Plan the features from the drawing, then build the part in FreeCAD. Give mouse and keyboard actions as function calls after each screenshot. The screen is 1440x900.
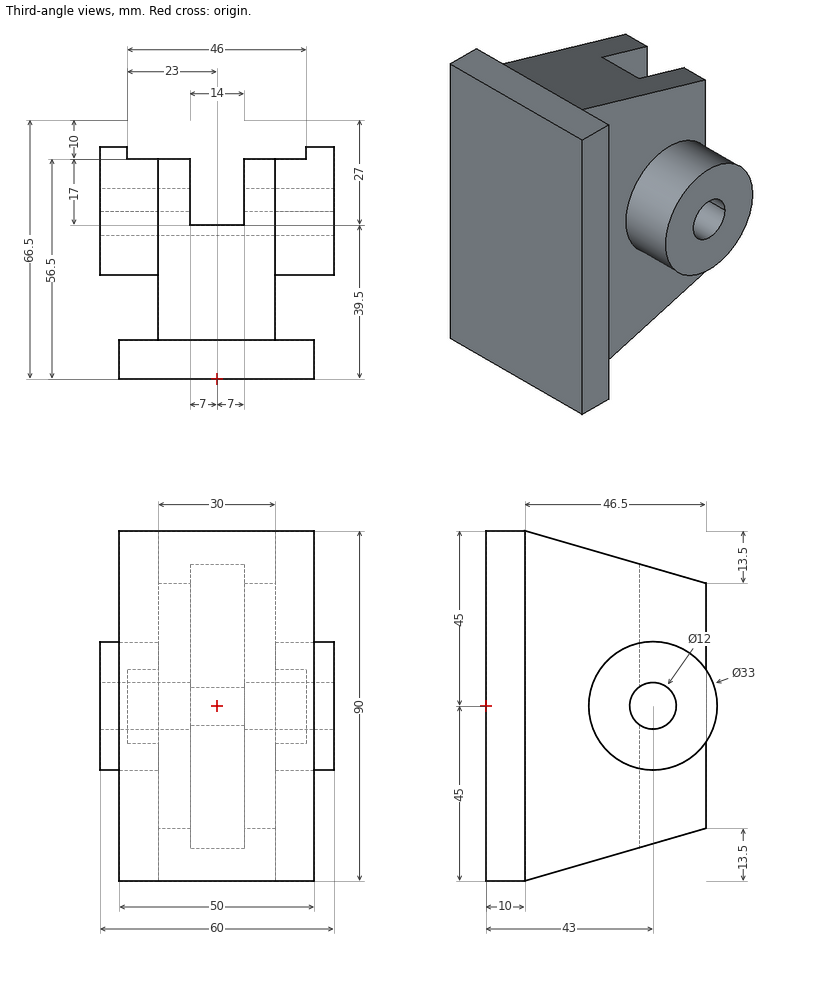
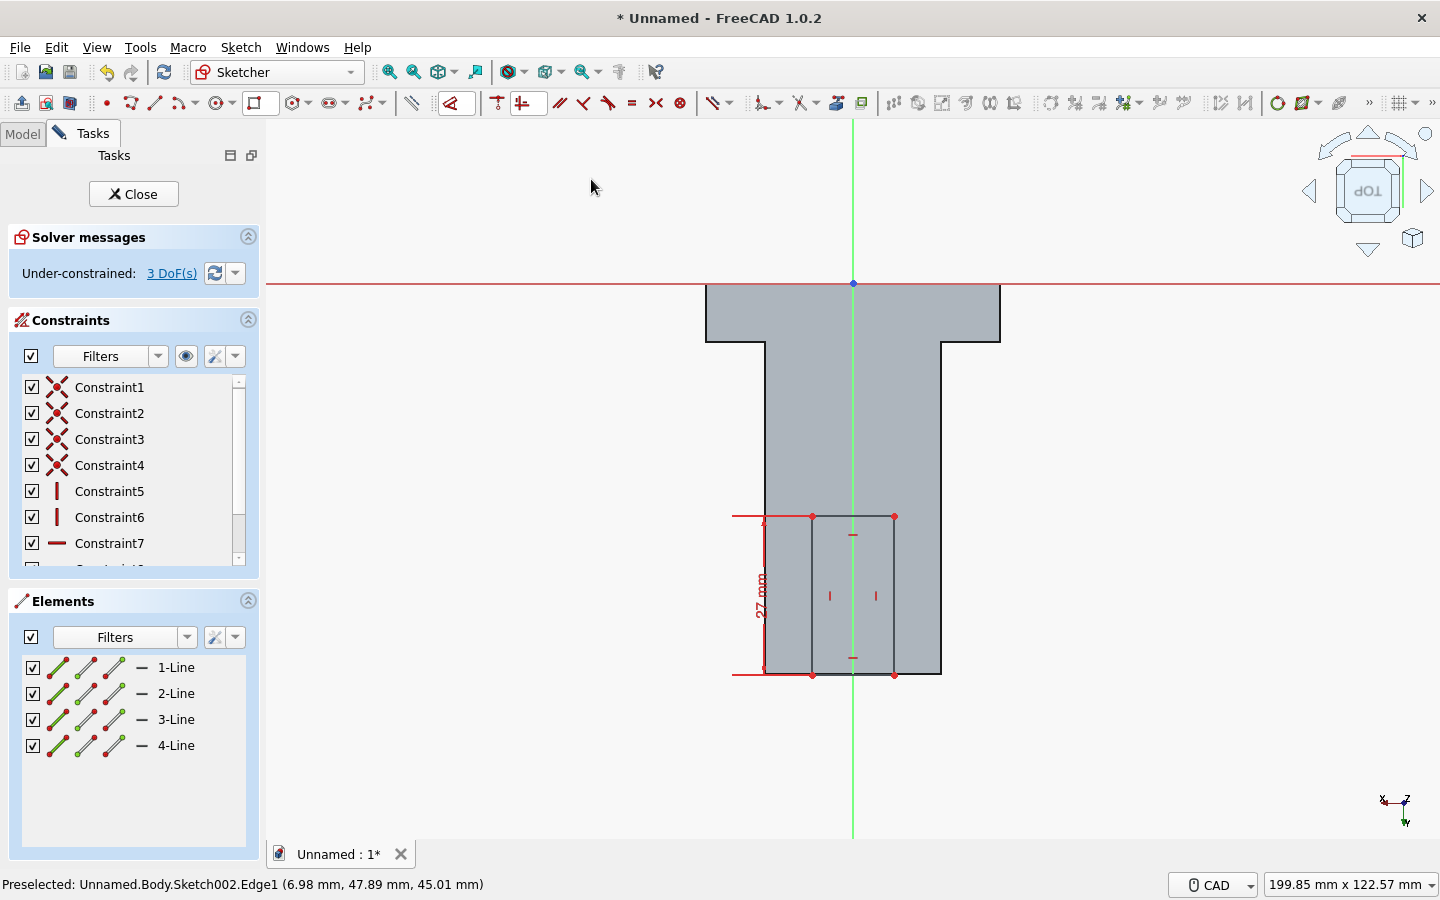
click(837, 675)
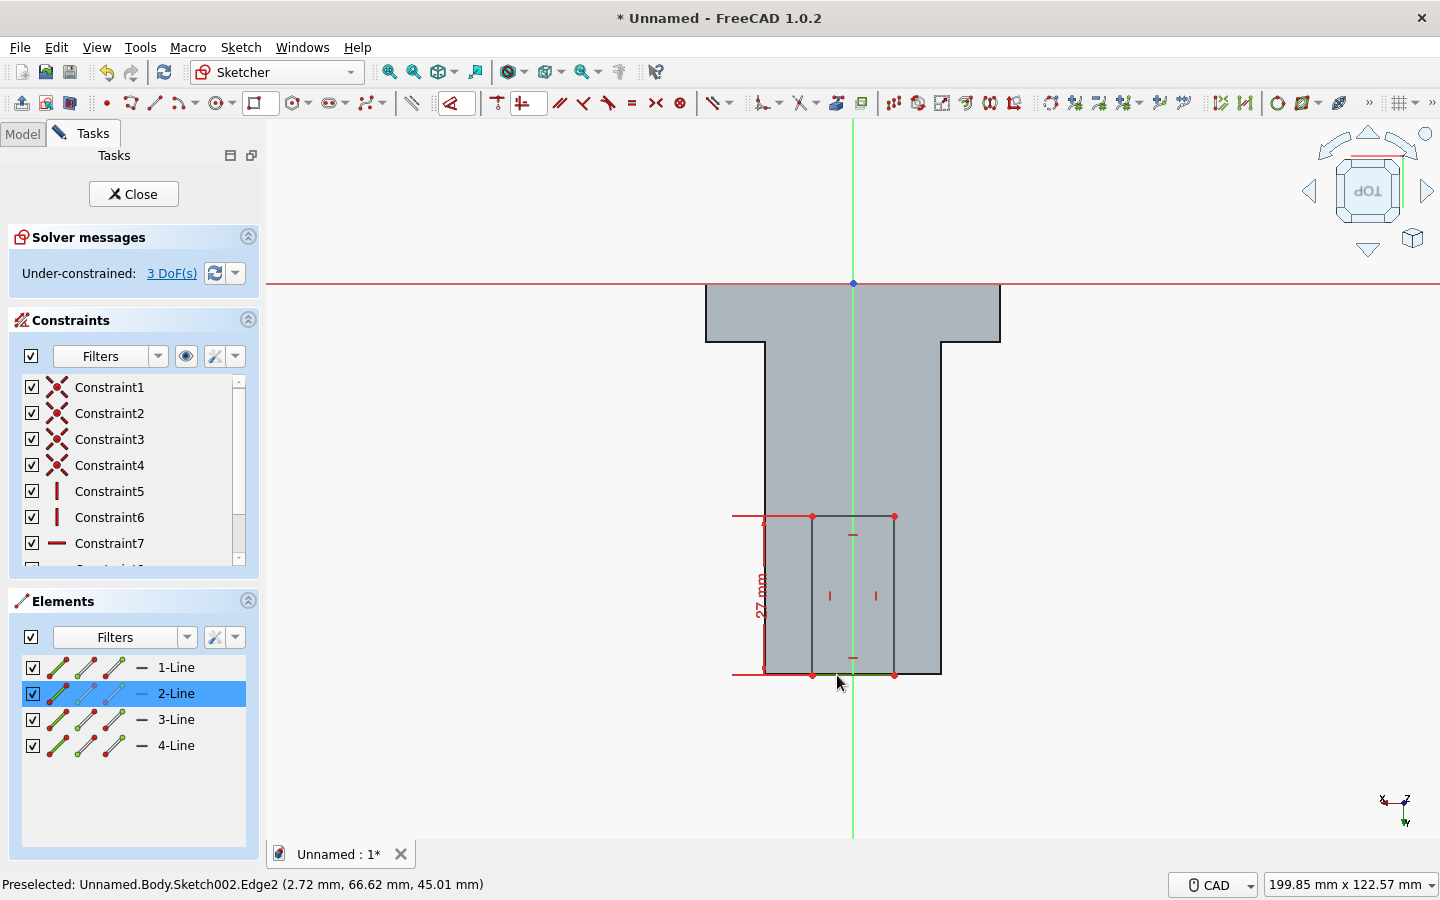
click(470, 104)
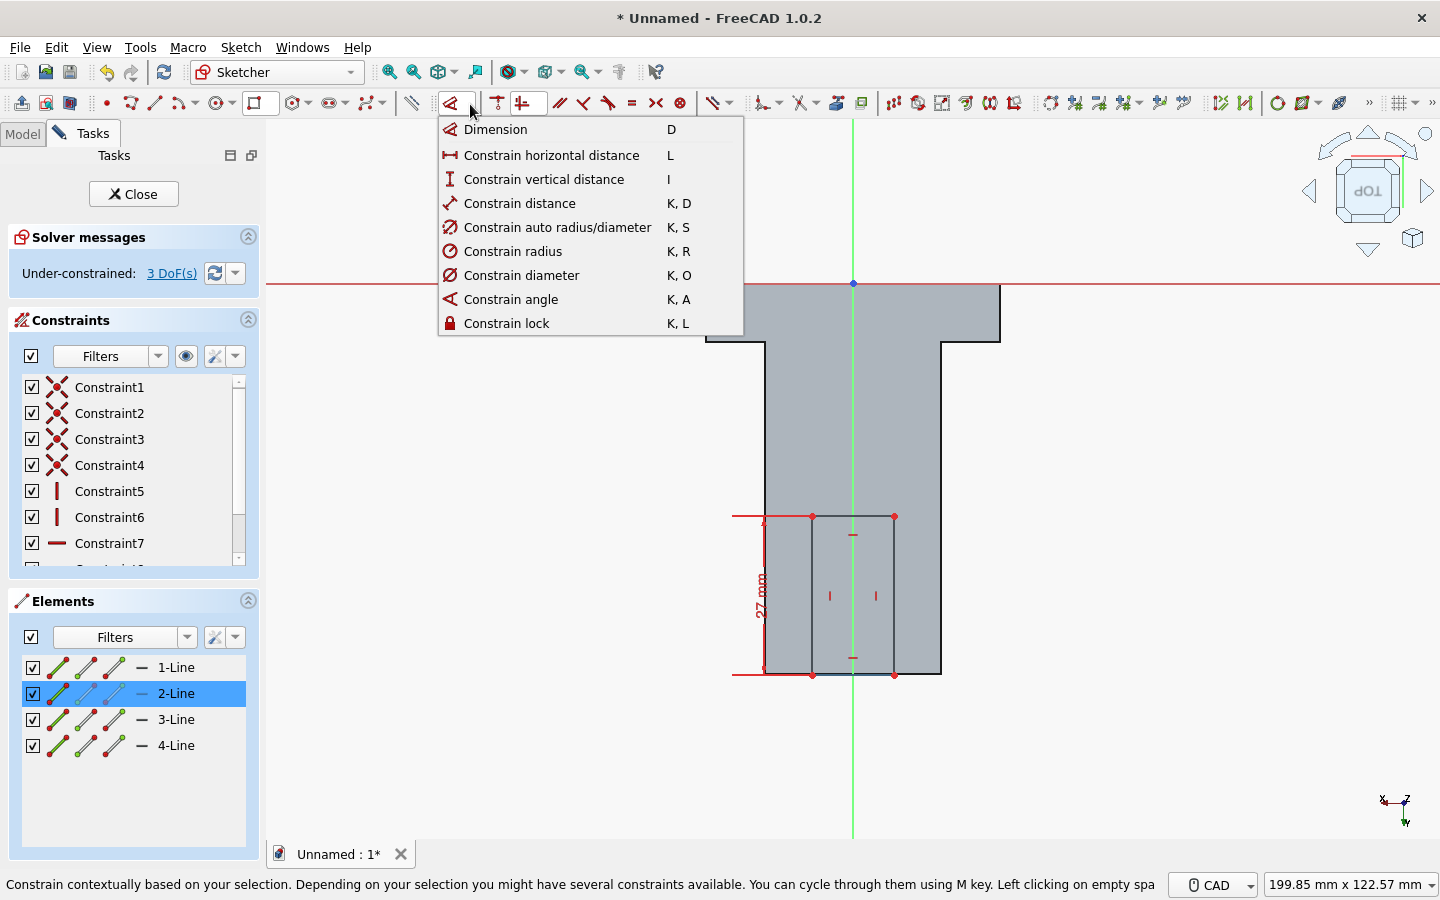
click(591, 155)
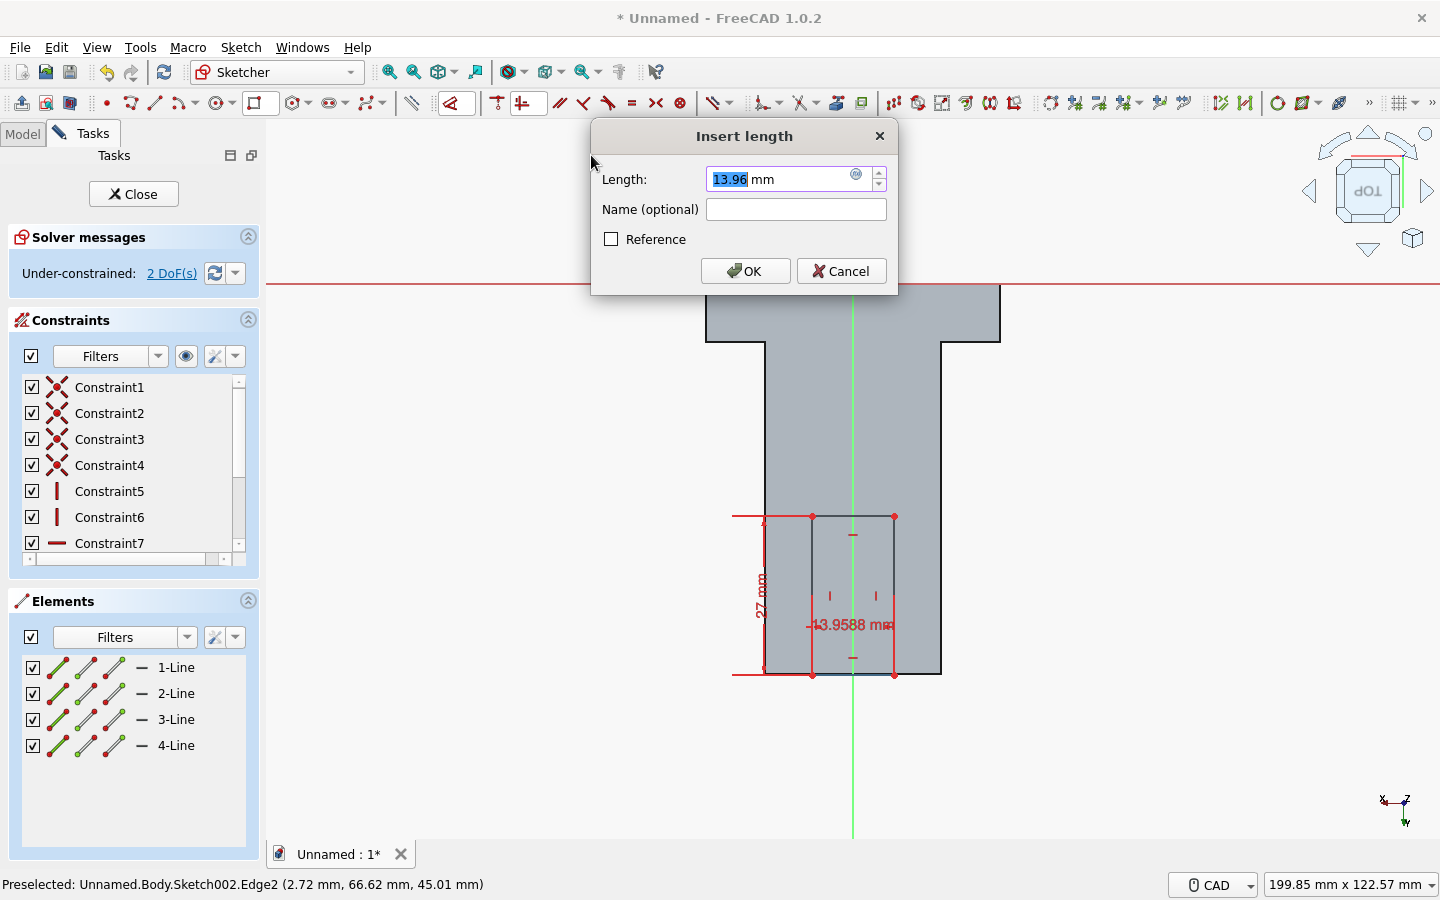
text(14)
key(Return)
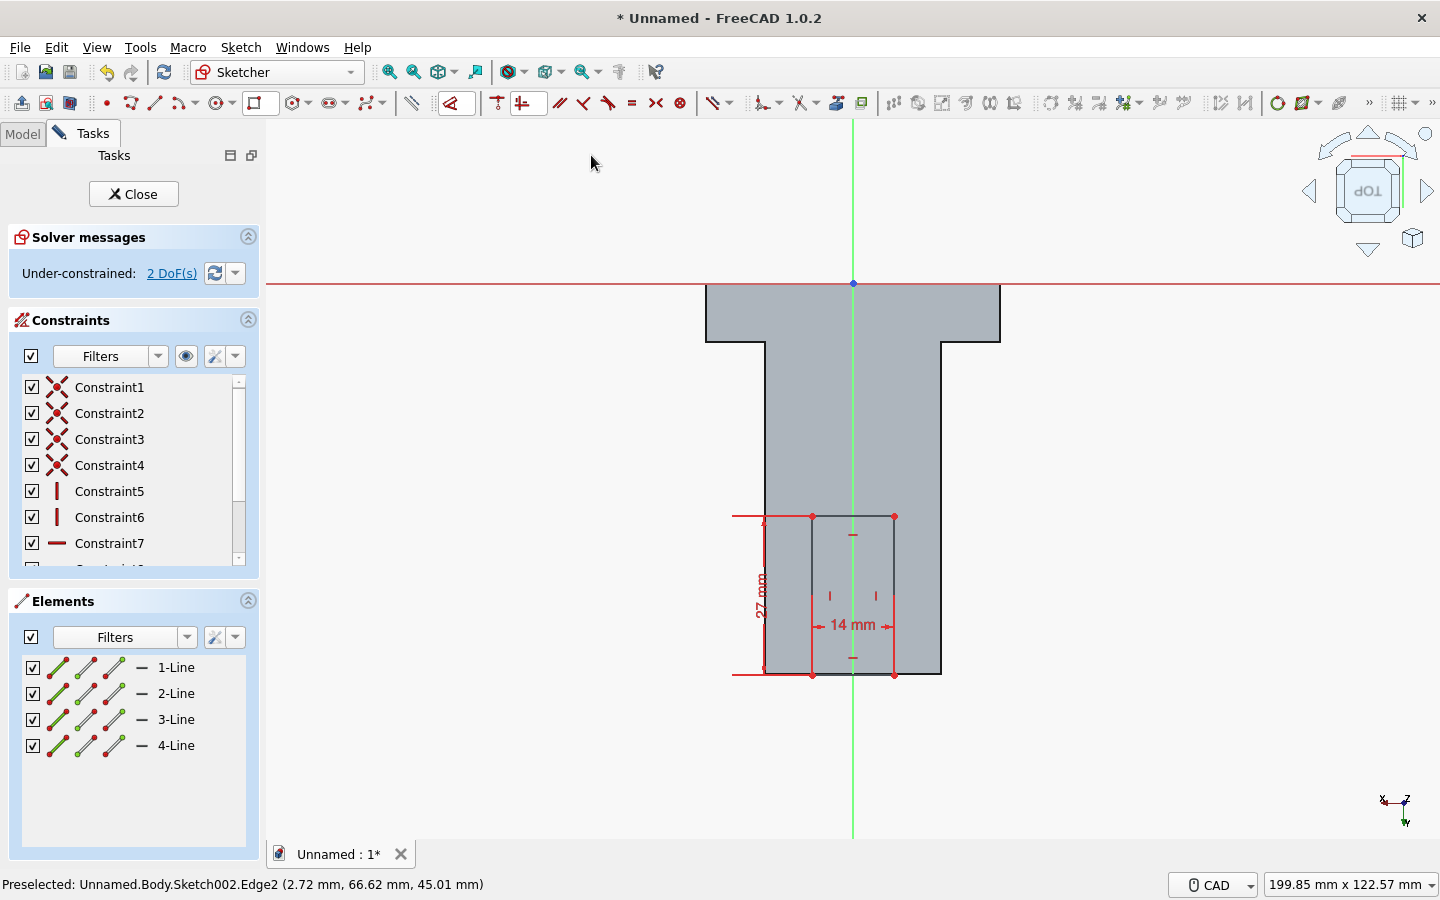
click(812, 516)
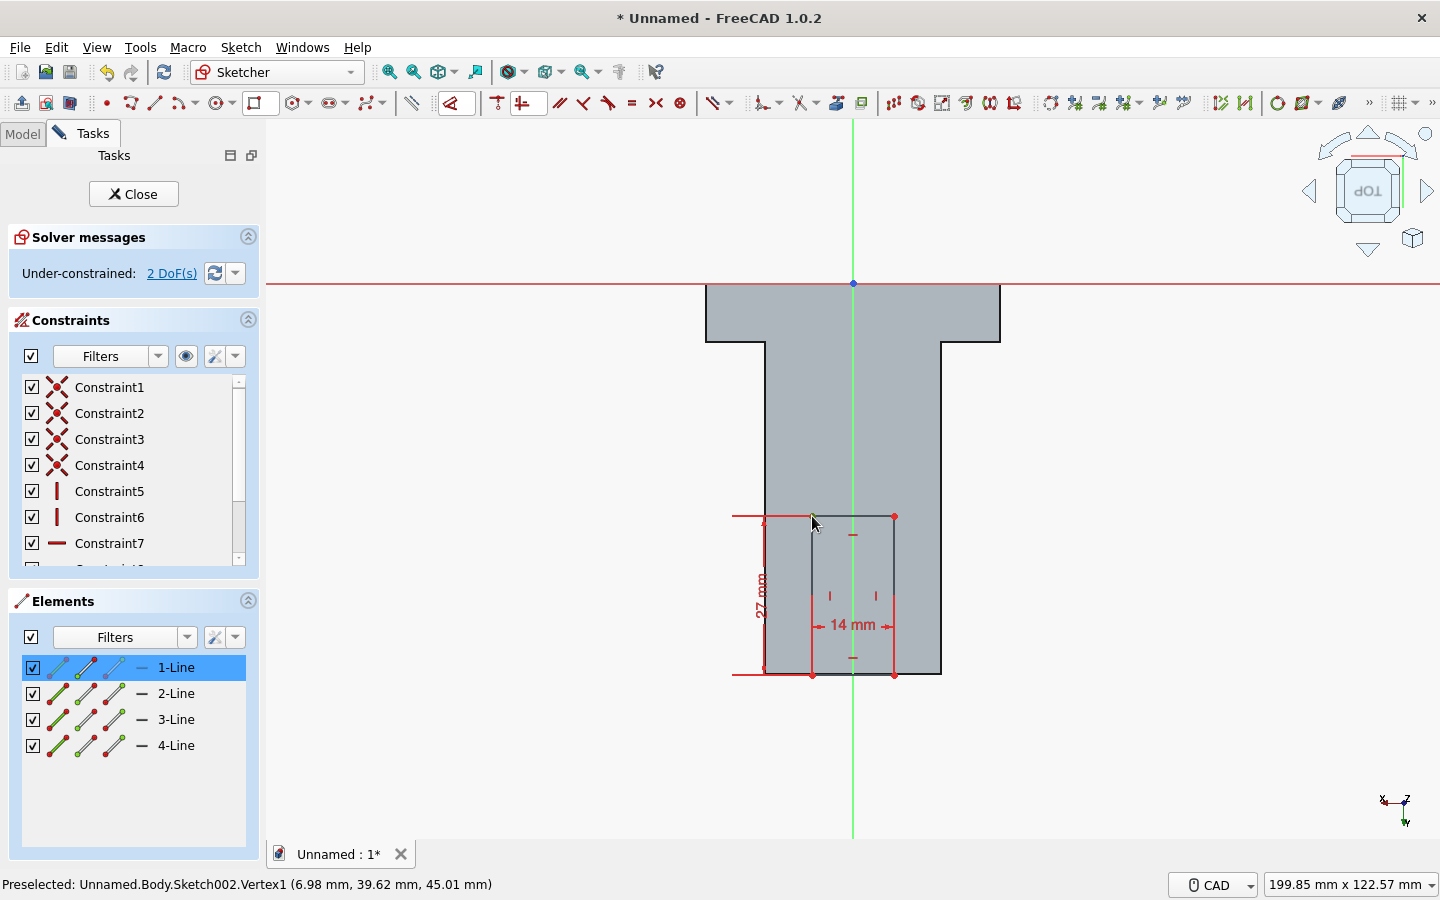
click(470, 104)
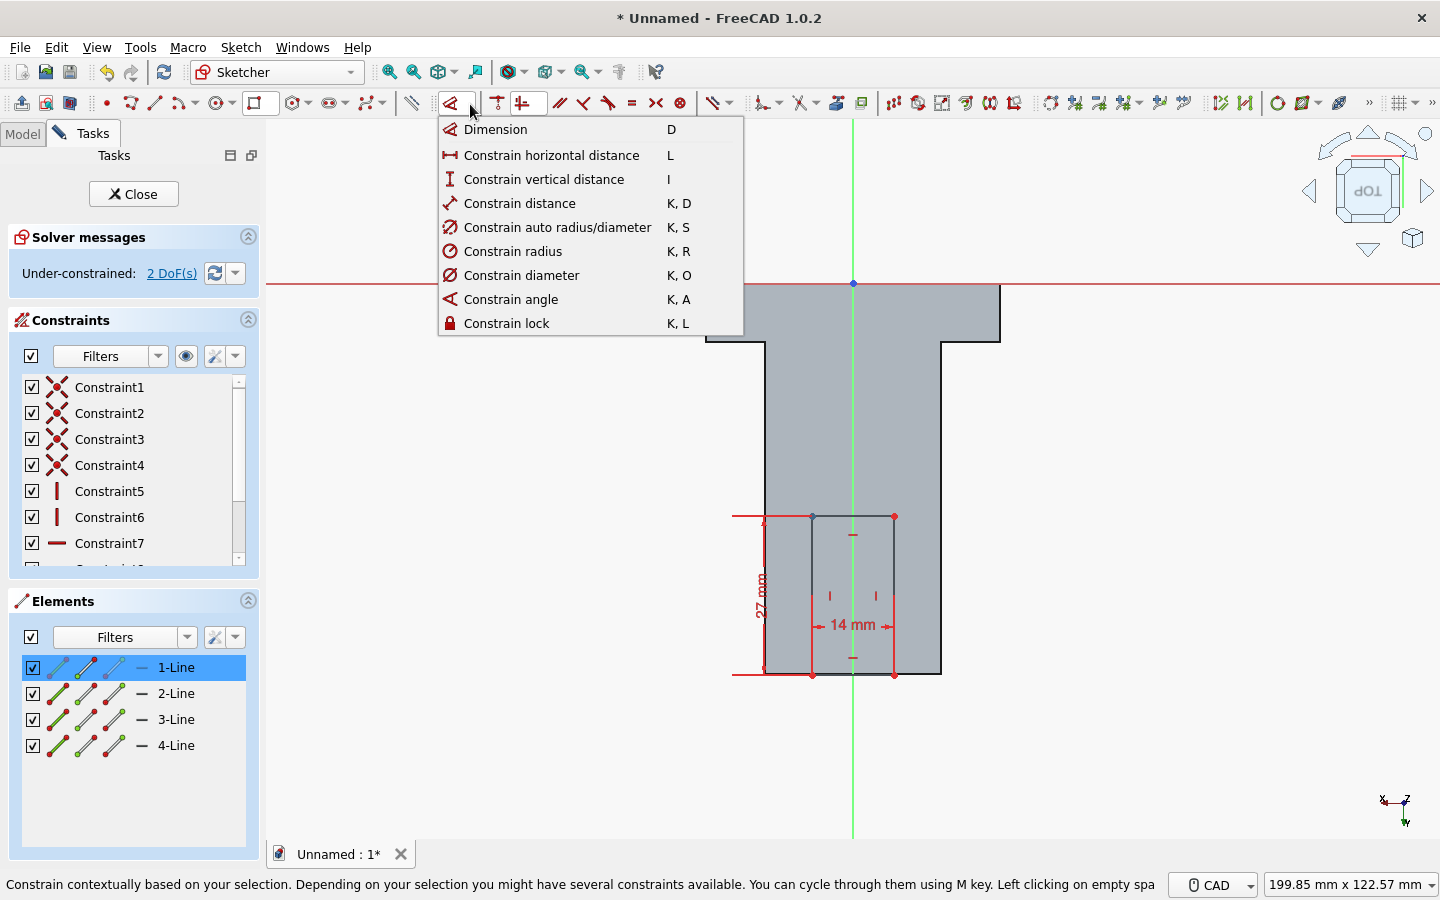
click(591, 155)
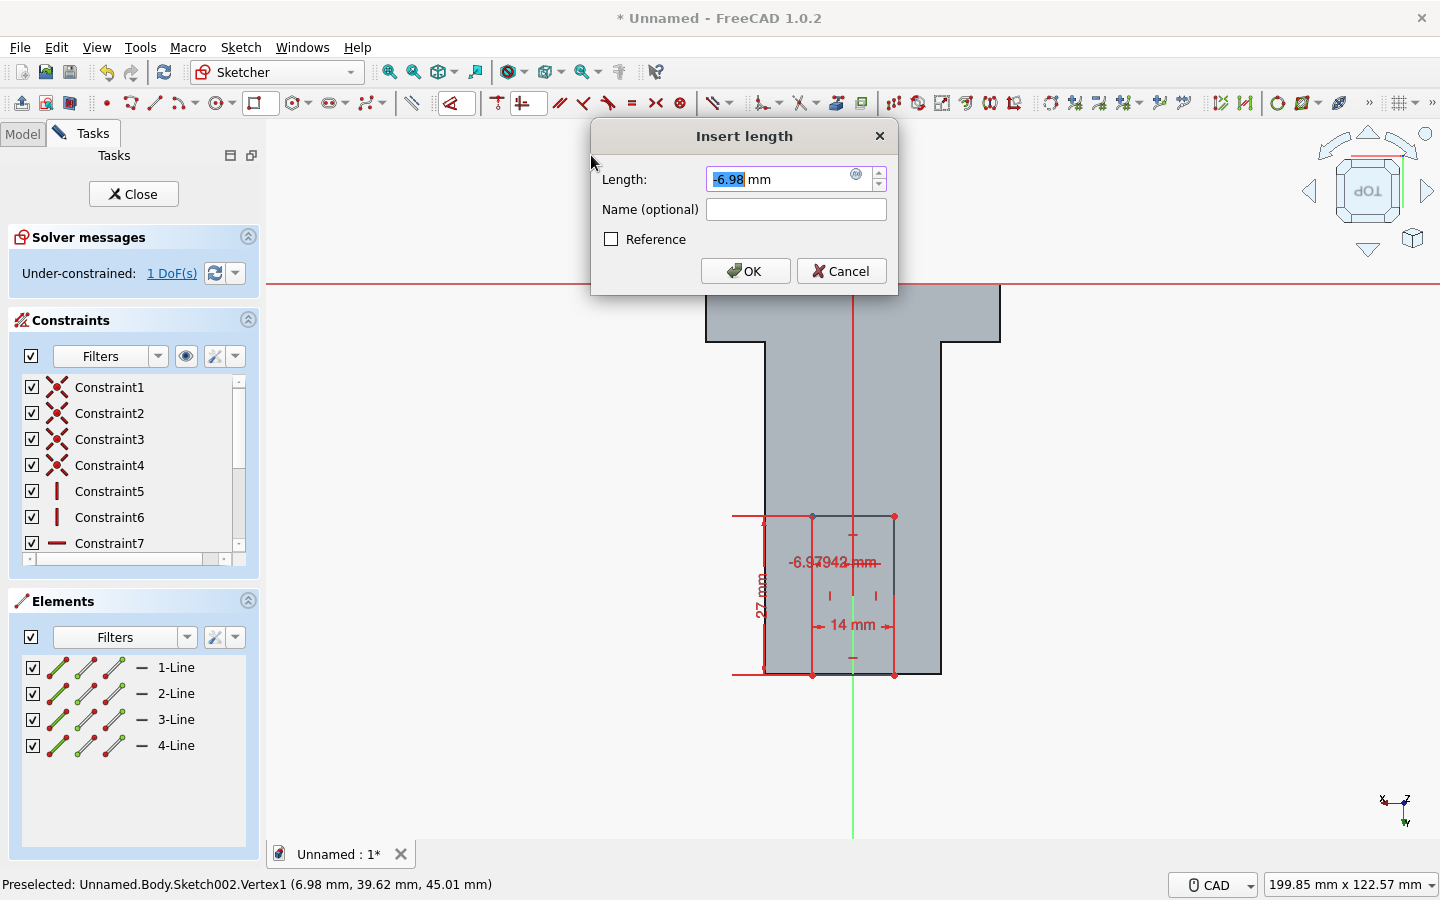
text(-7)
key(Return)